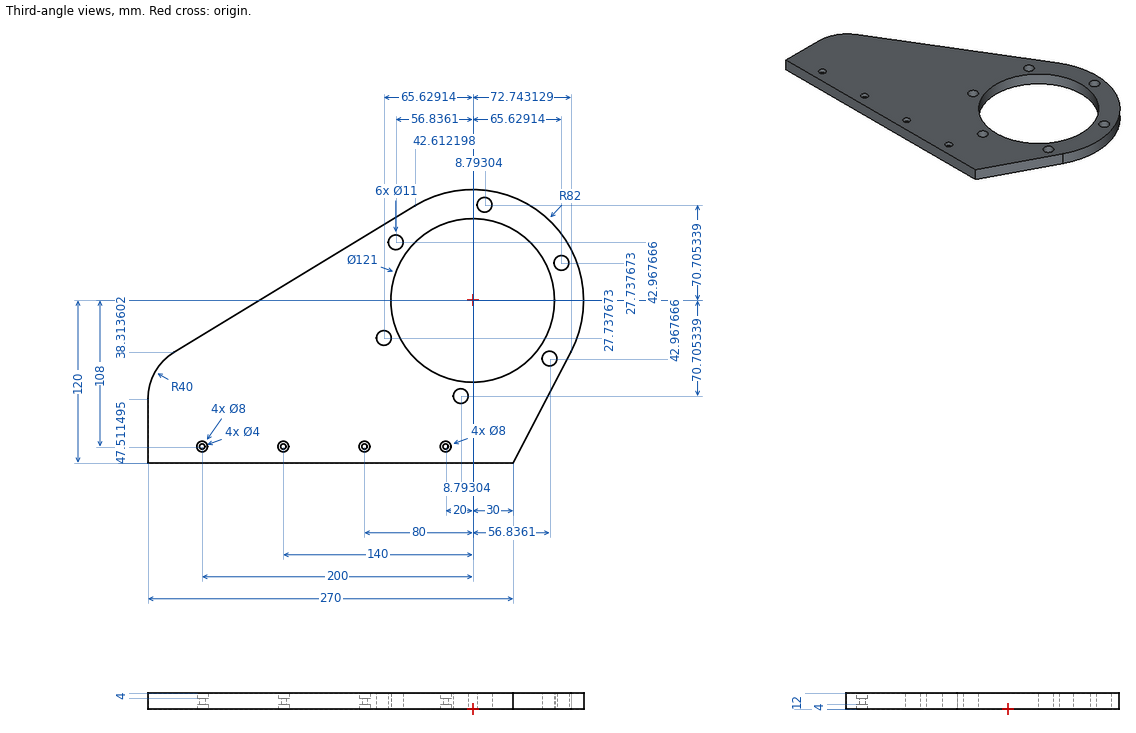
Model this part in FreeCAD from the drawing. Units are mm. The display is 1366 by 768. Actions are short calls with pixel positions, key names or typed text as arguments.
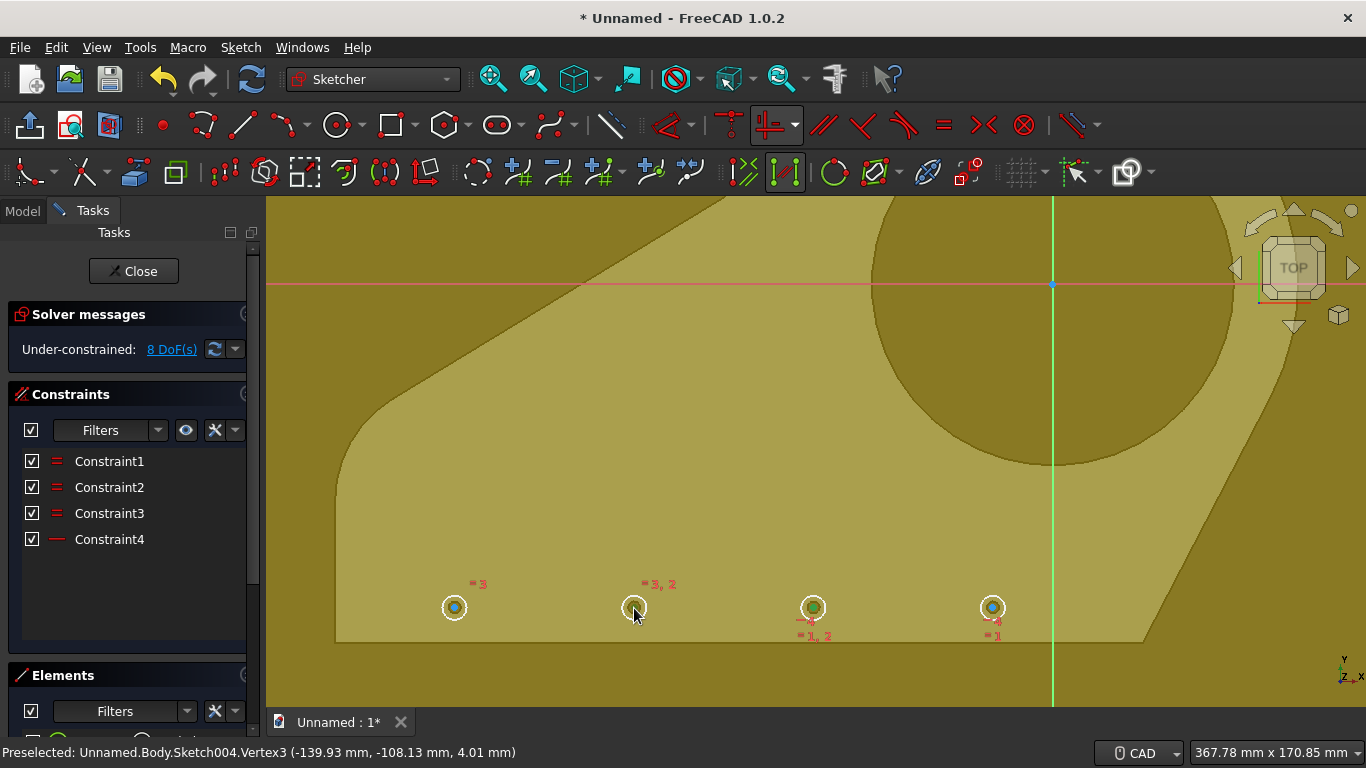
key(h)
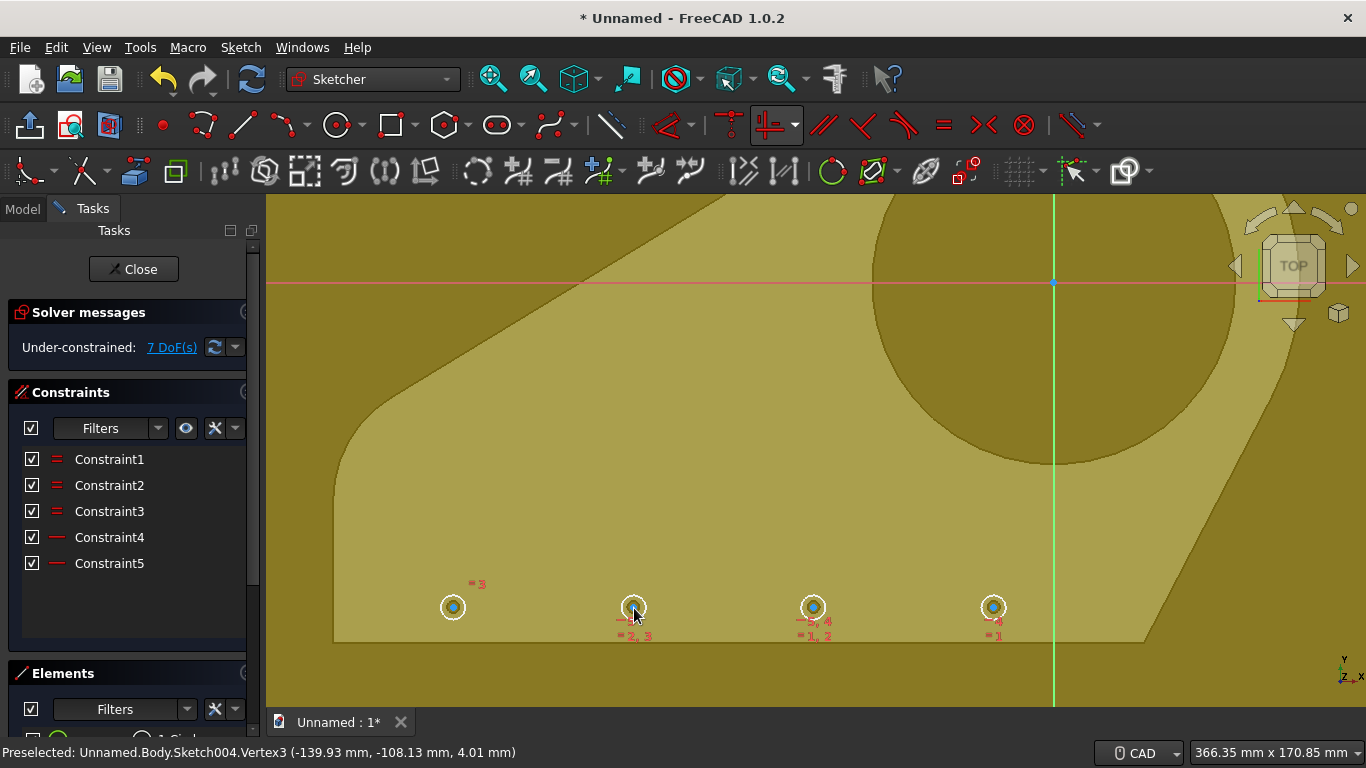
click(634, 608)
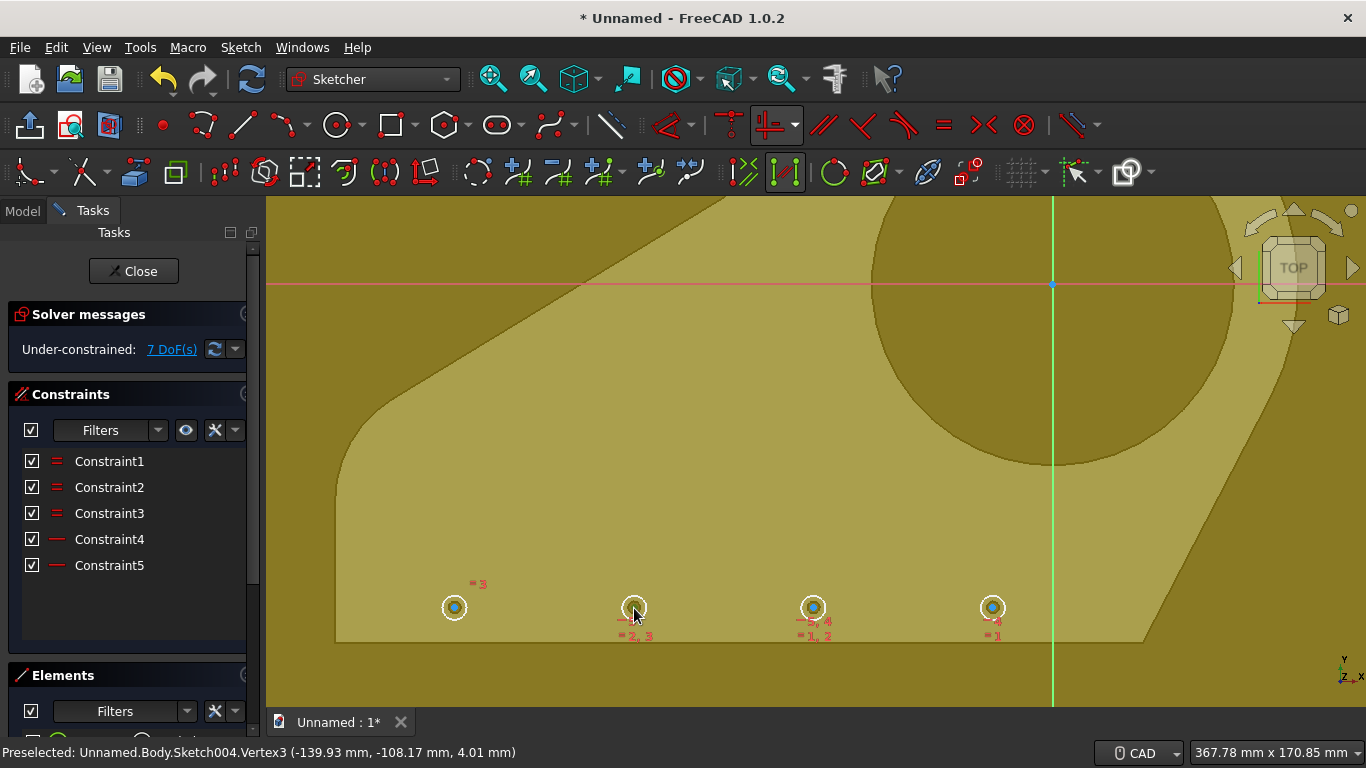
click(455, 608)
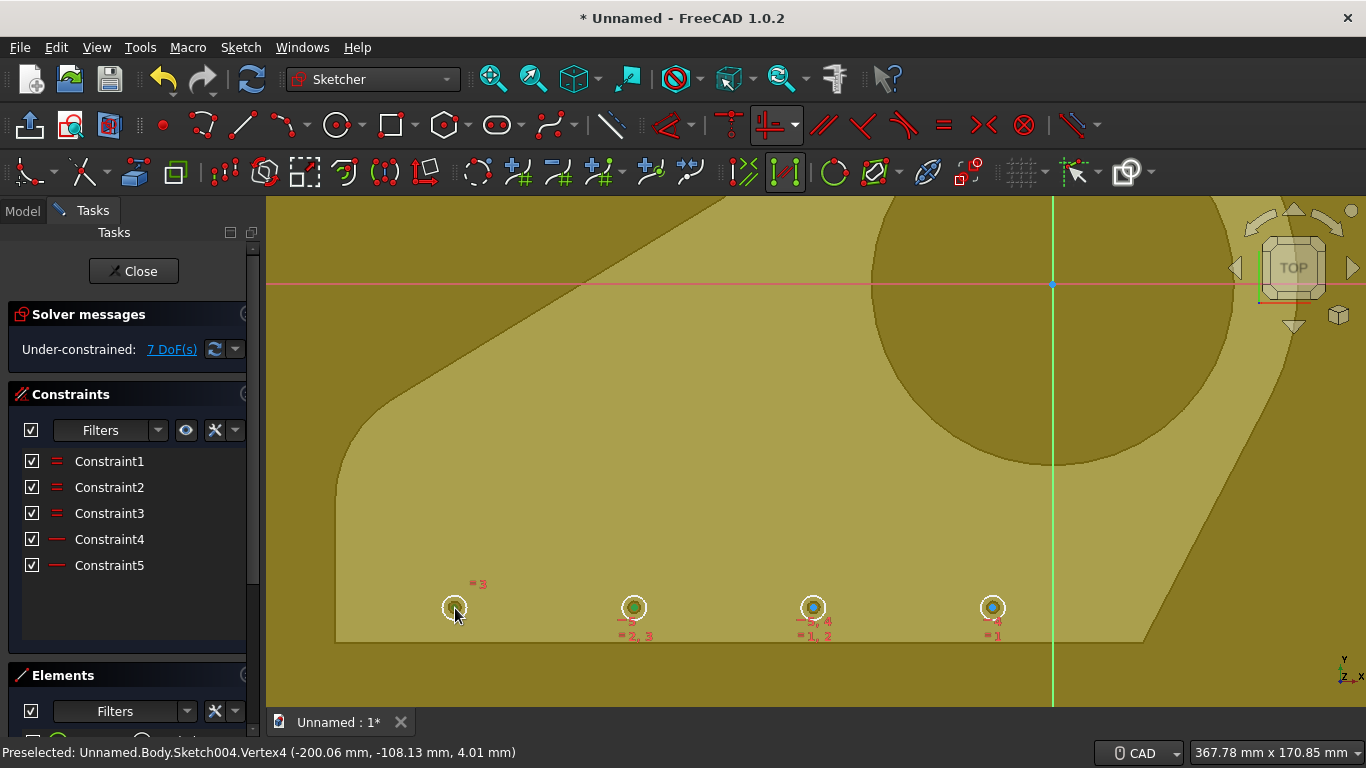
key(h)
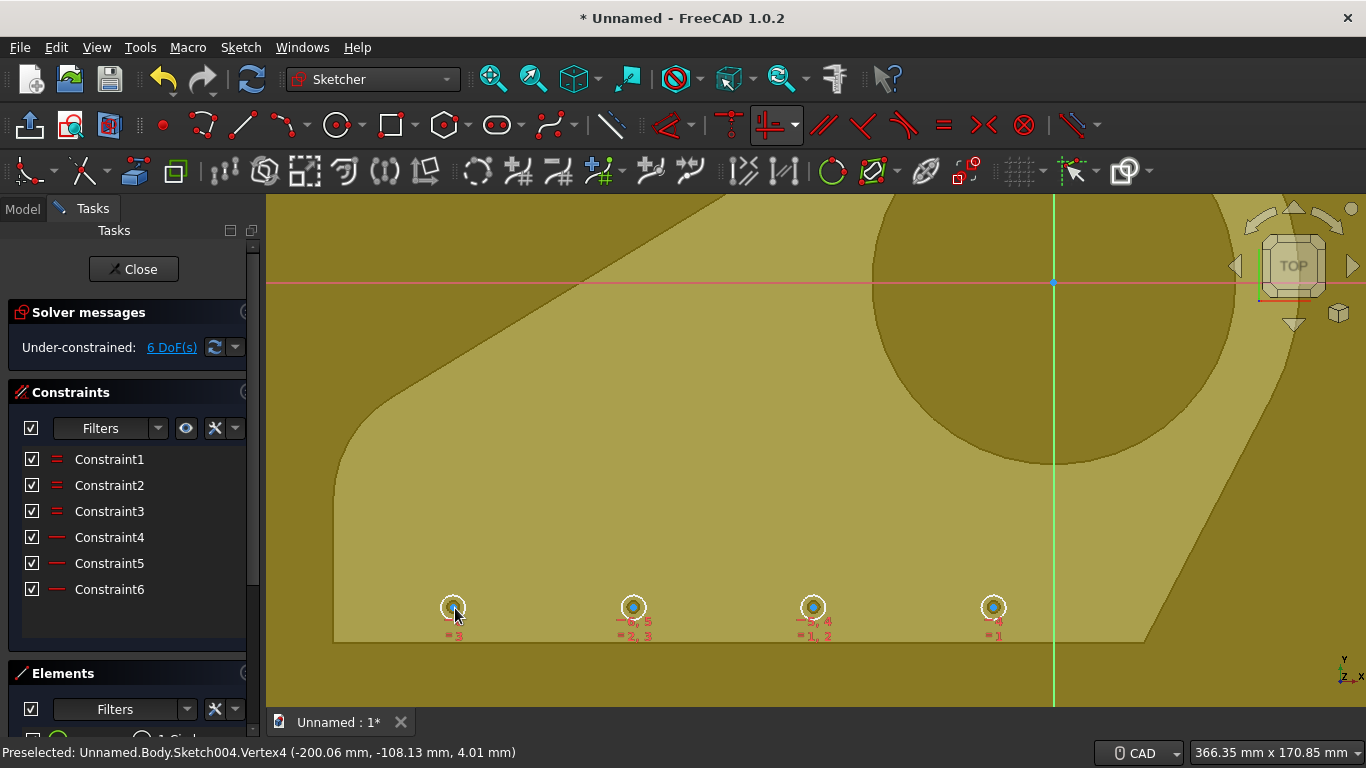
click(666, 126)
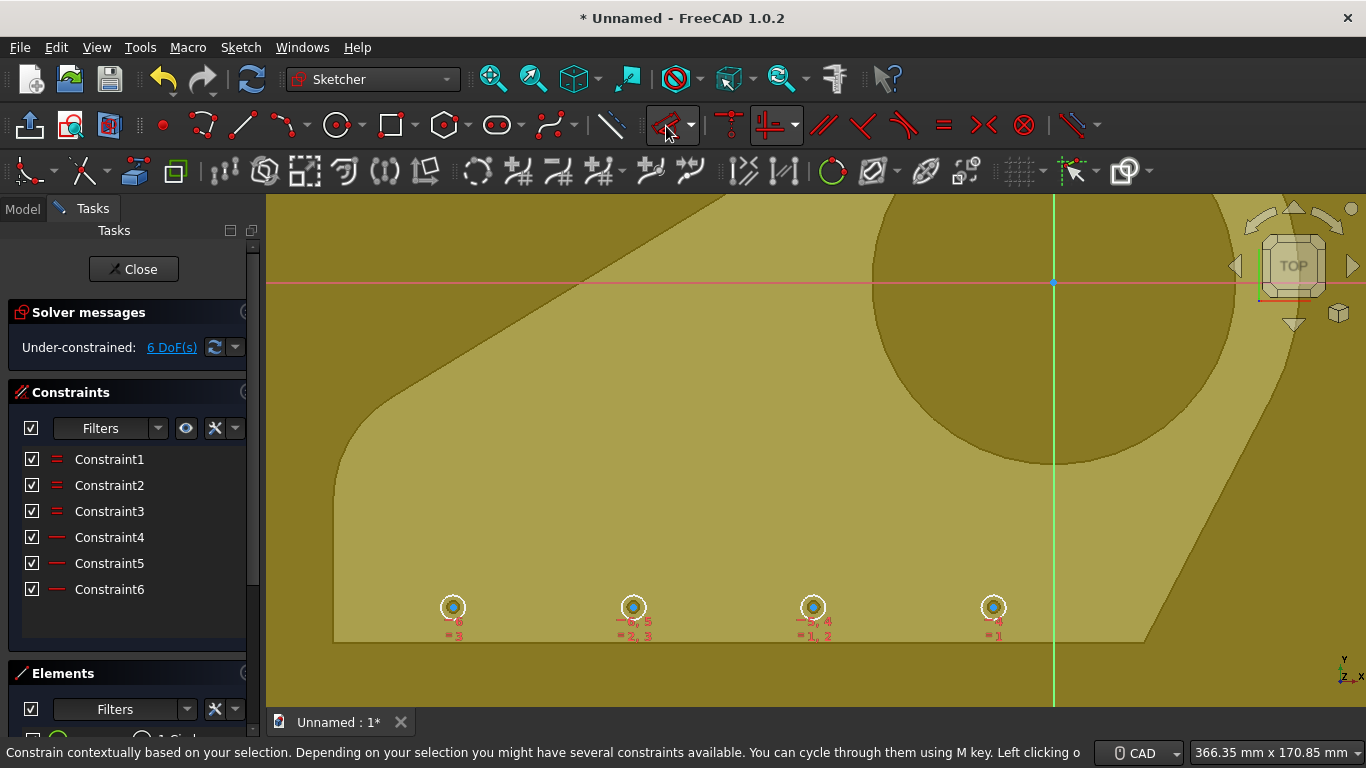
scroll(1002, 599, up, 3)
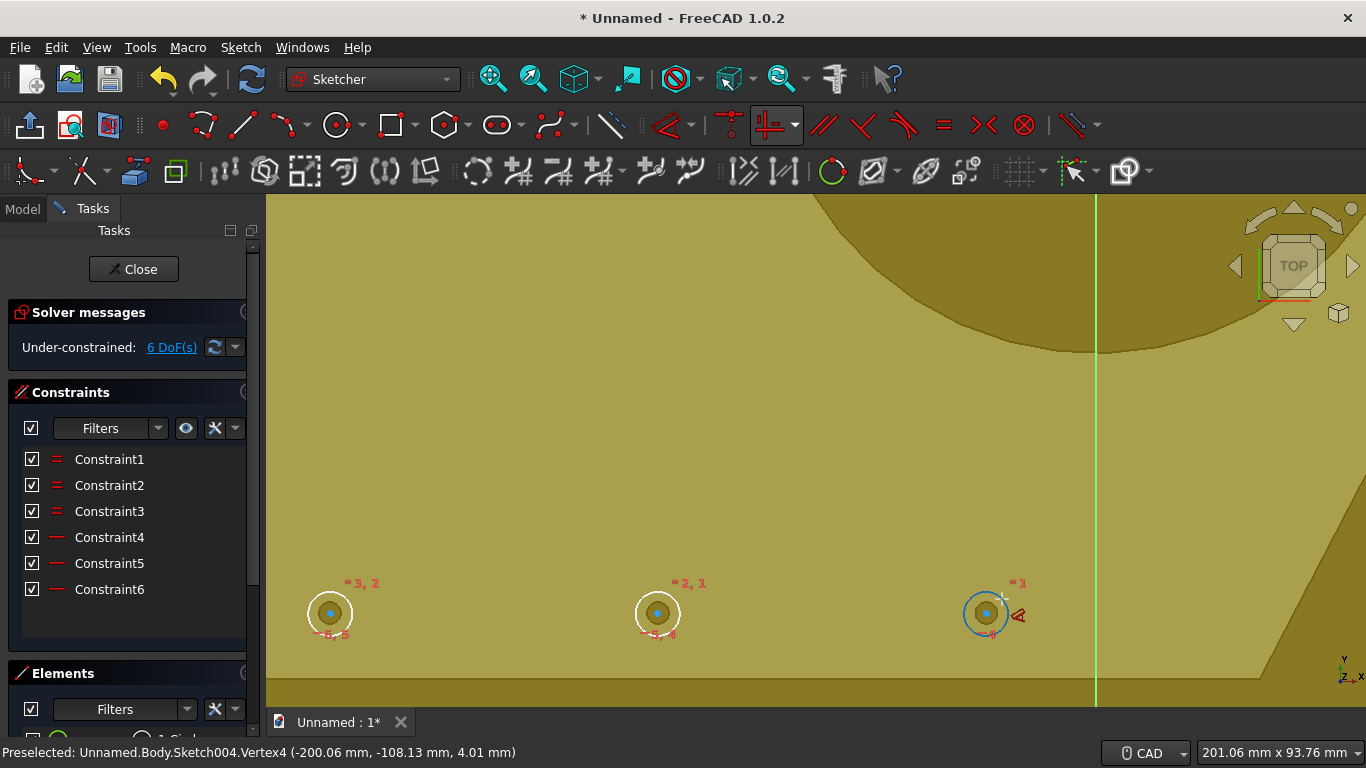
click(1002, 598)
click(1025, 575)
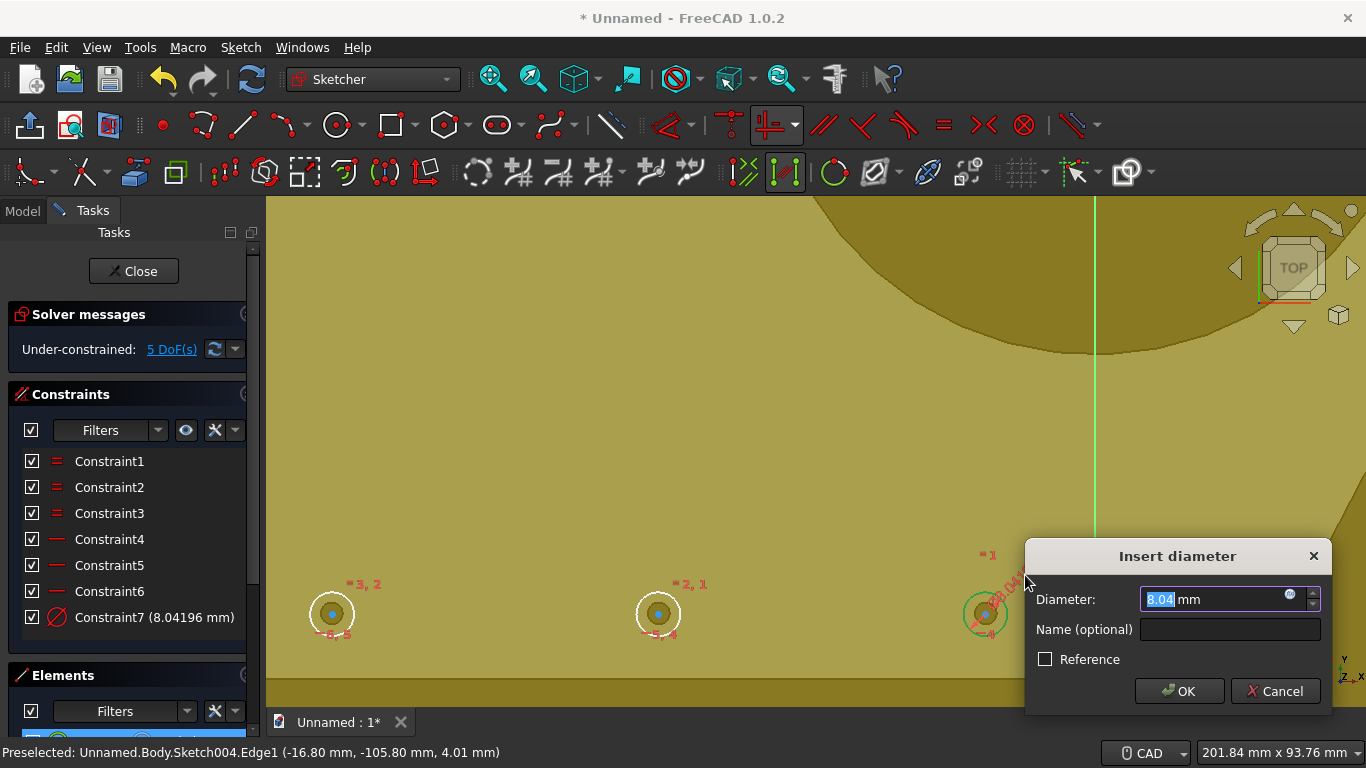
text(8)
key(Return)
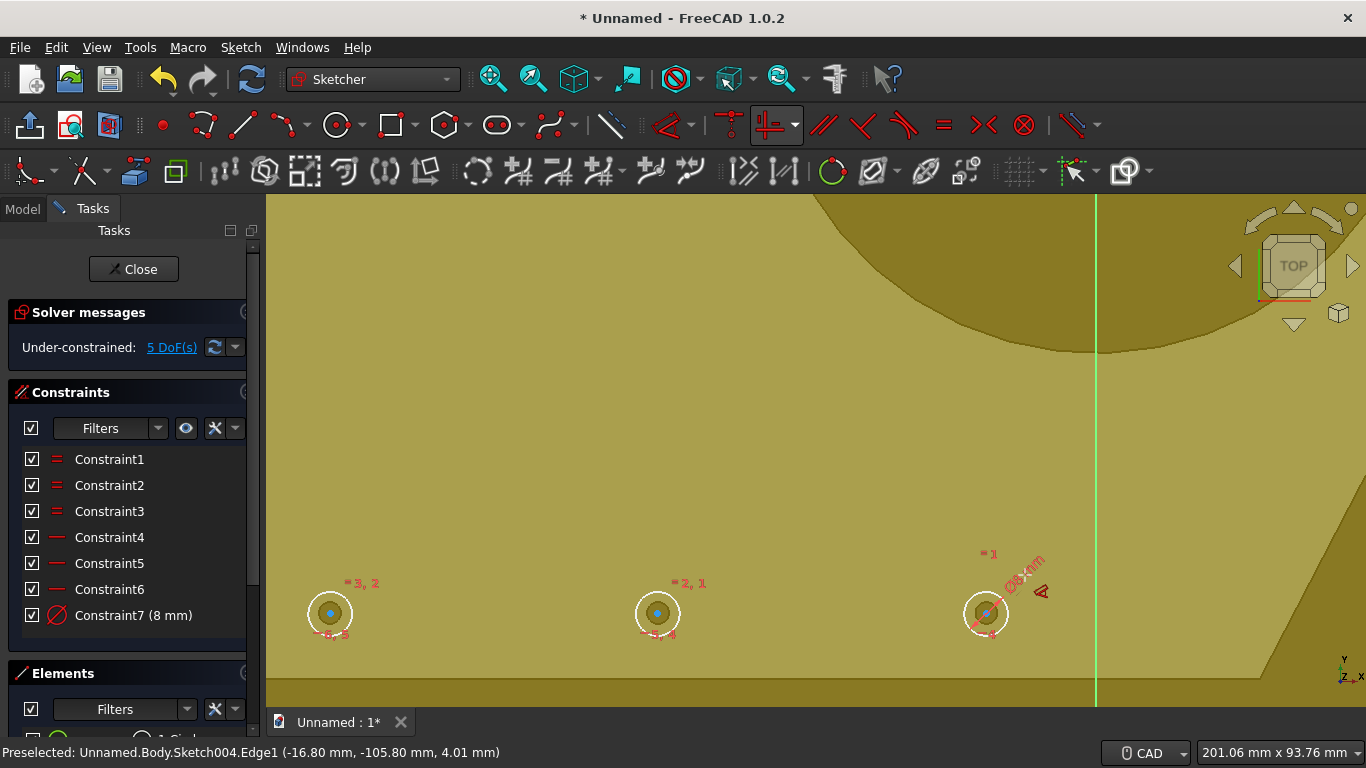
click(986, 614)
click(1041, 648)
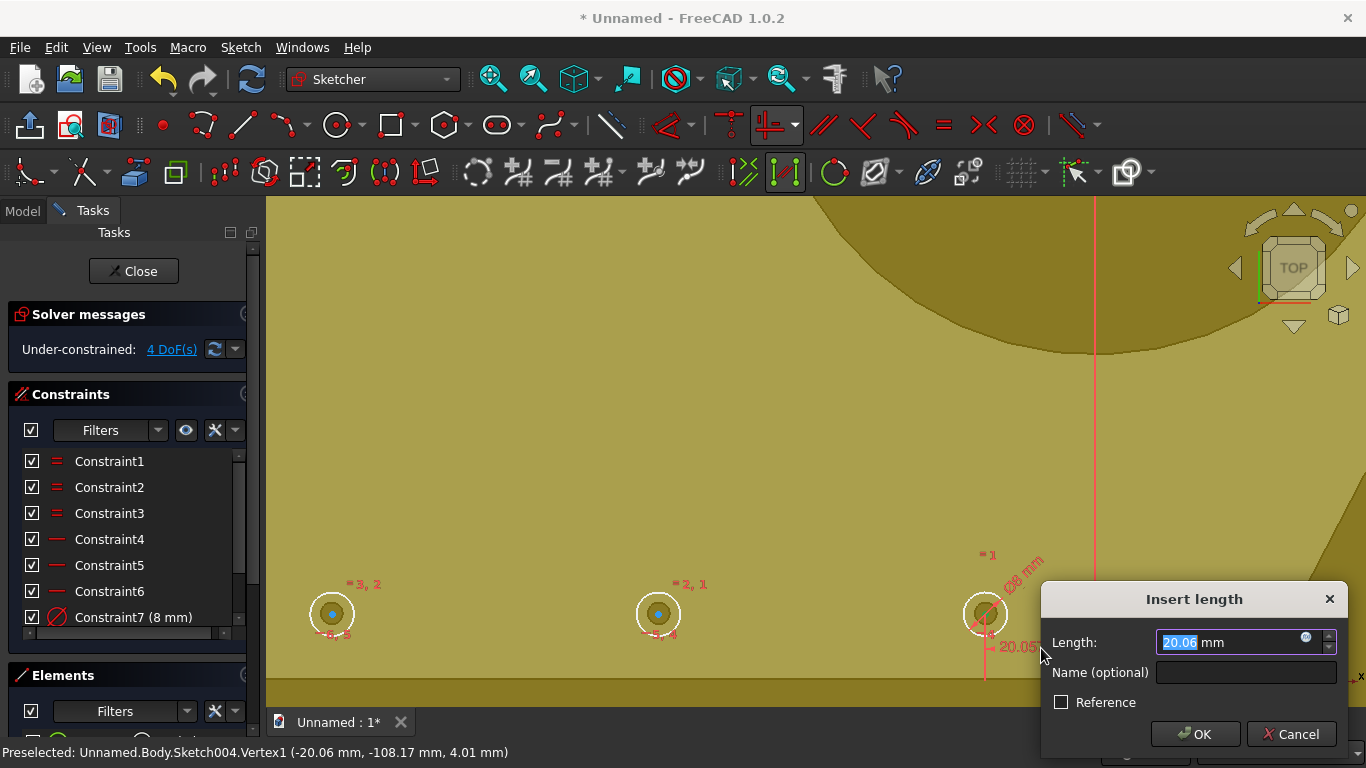
text(20)
key(Return)